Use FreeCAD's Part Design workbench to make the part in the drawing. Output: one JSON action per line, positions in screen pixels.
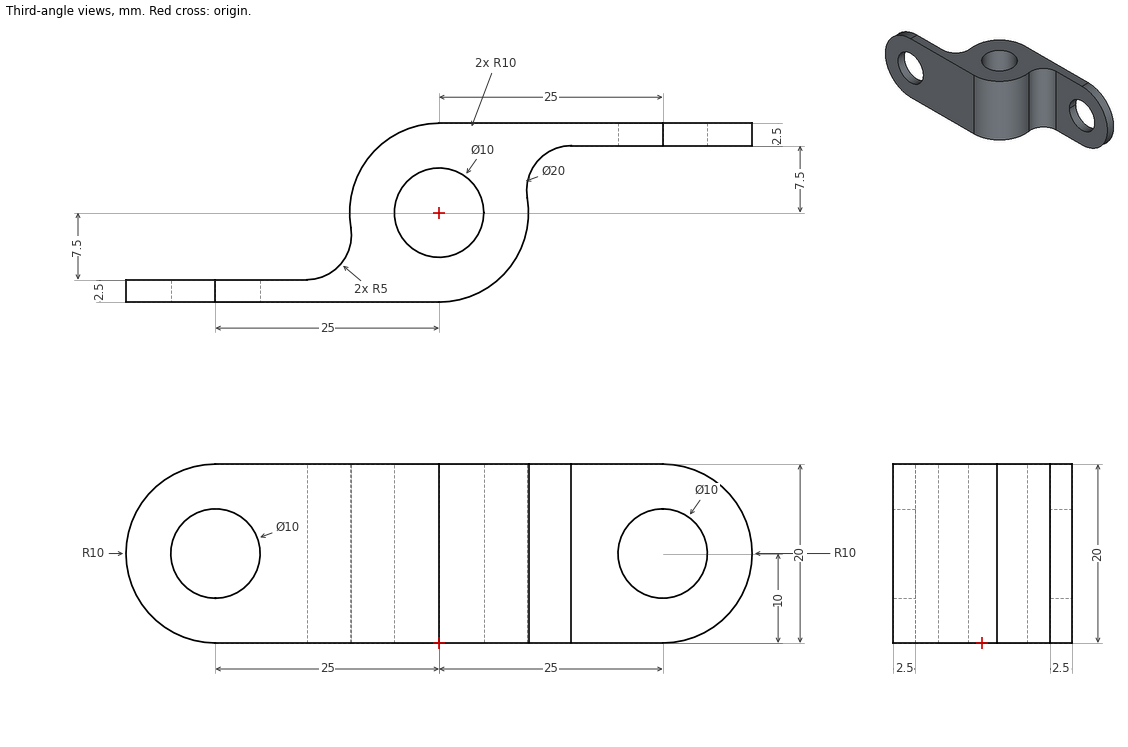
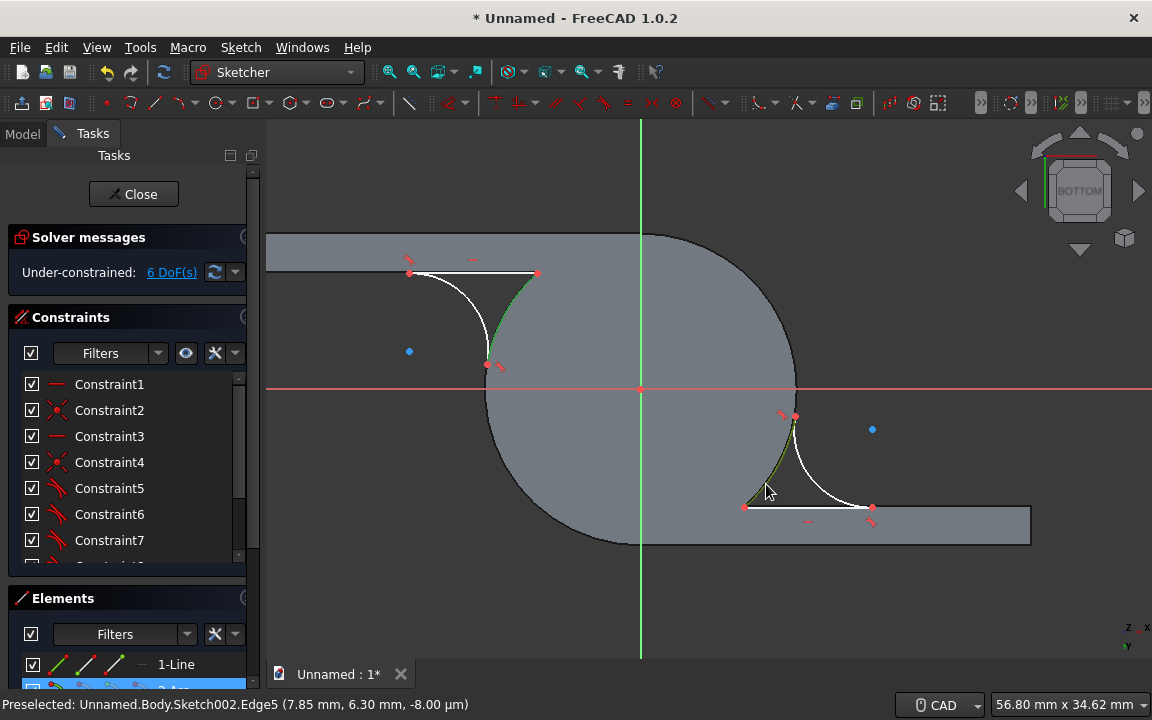
{"action": "key", "text": "e"}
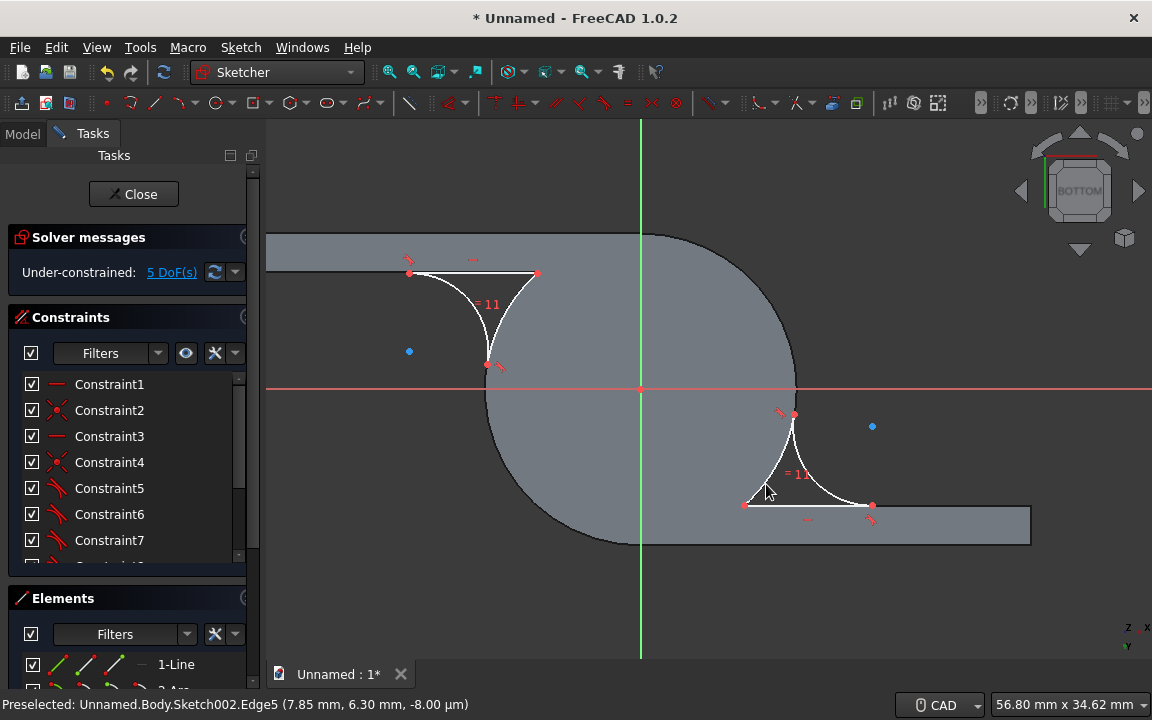
{"action": "left_click", "coordinate": [483, 324]}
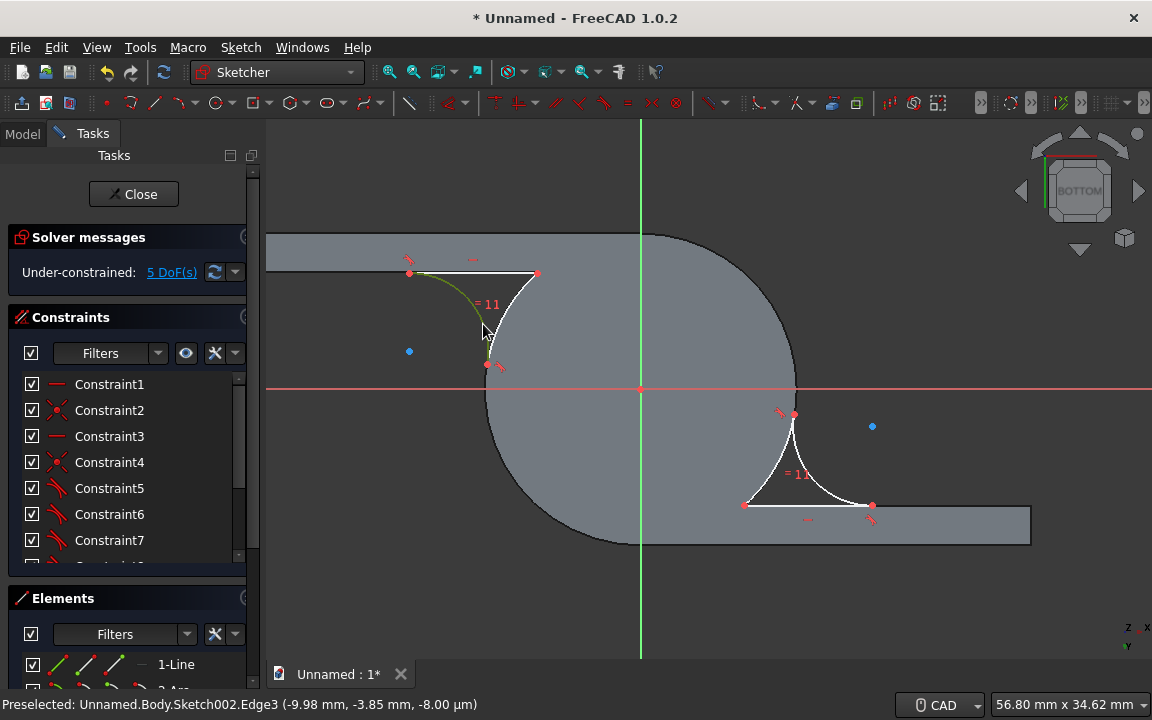
{"action": "left_click", "coordinate": [798, 455]}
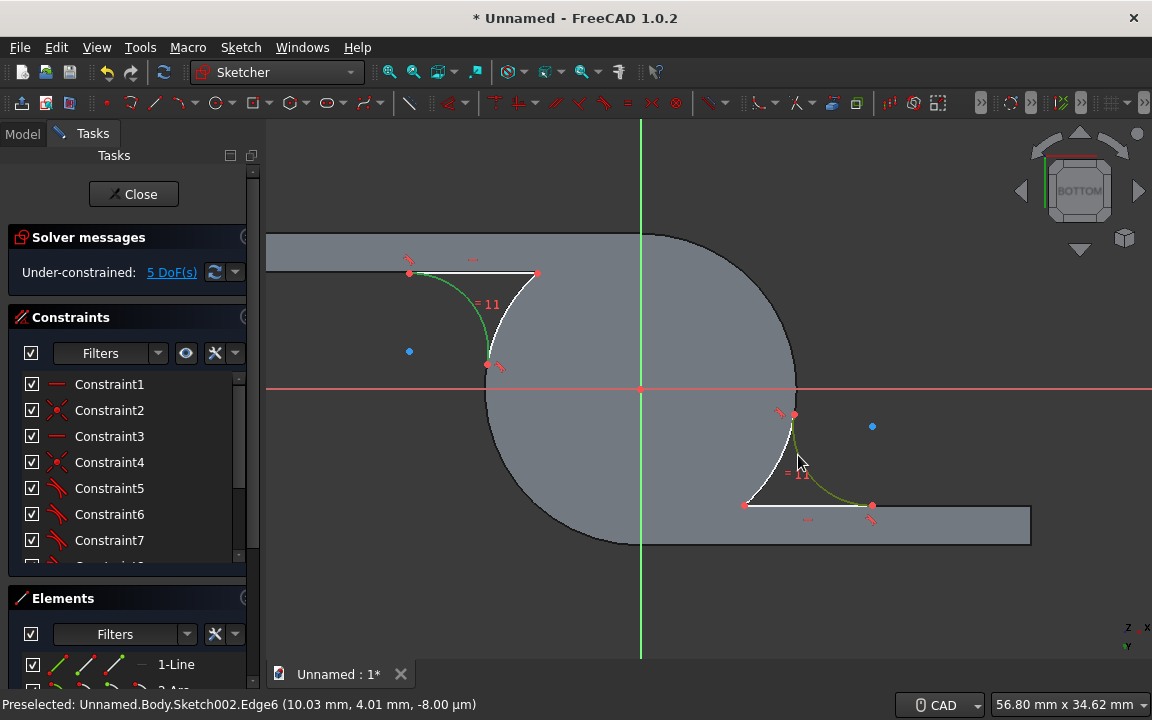
{"action": "key", "text": "e"}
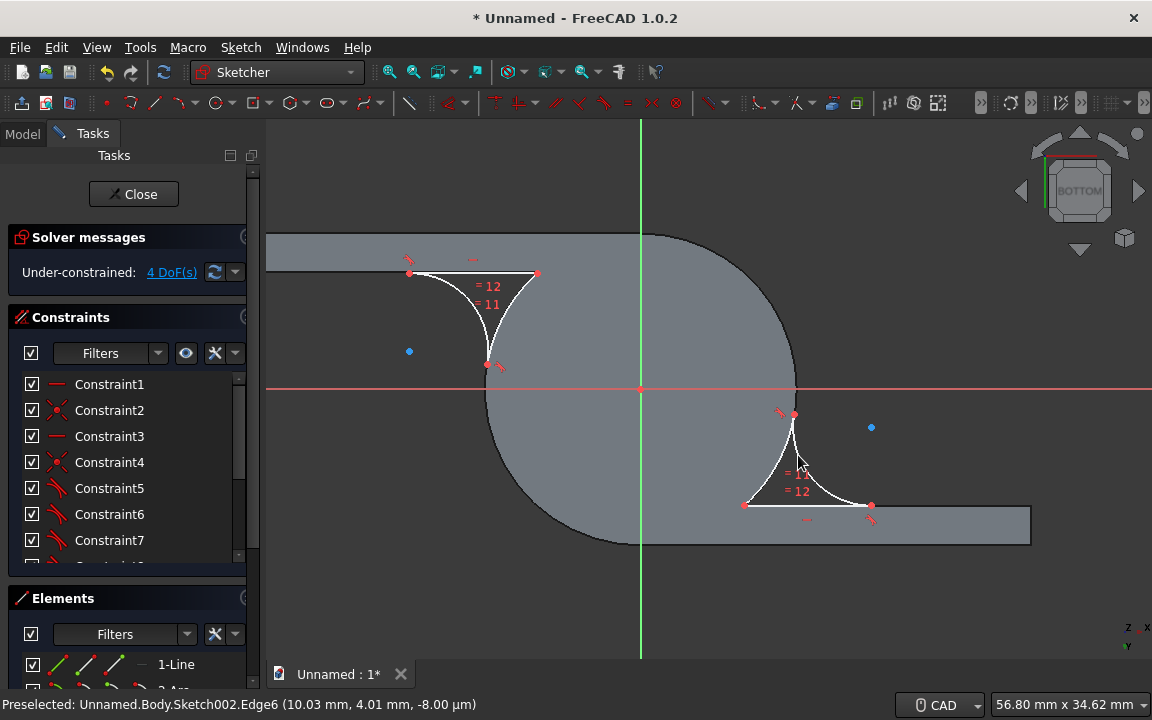
{"action": "left_click", "coordinate": [448, 104]}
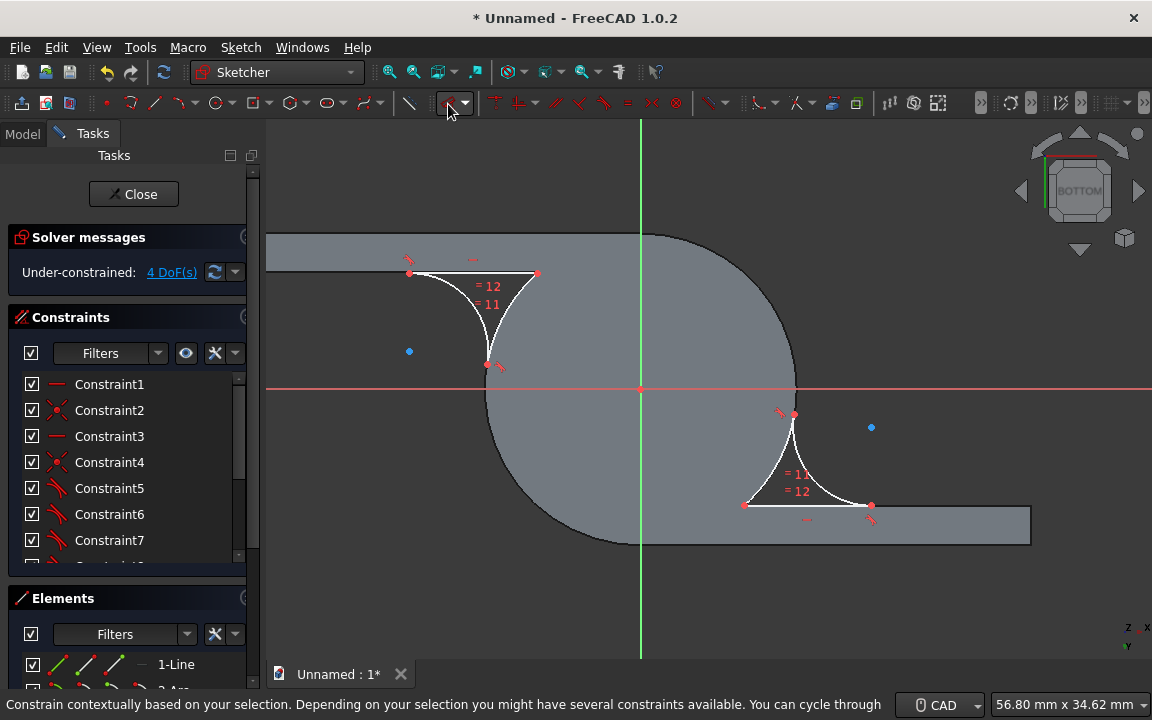
{"action": "left_click", "coordinate": [516, 297]}
{"action": "left_click", "coordinate": [562, 219]}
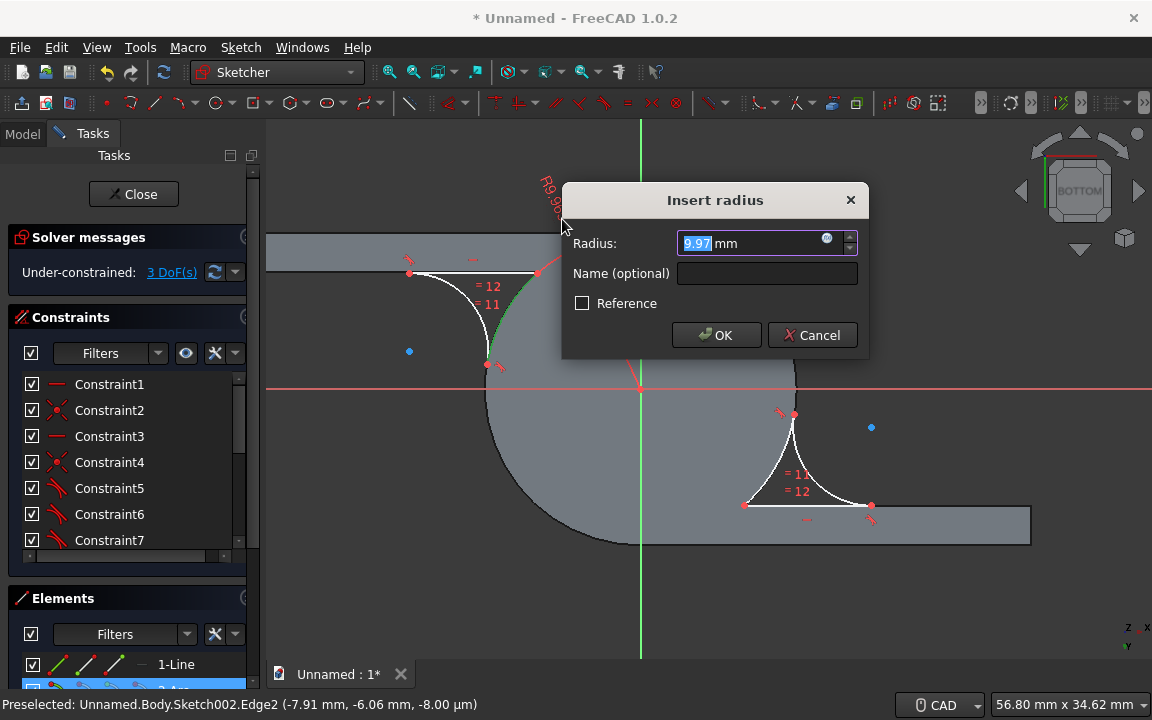
{"action": "type", "text": "10"}
{"action": "key", "text": "Return"}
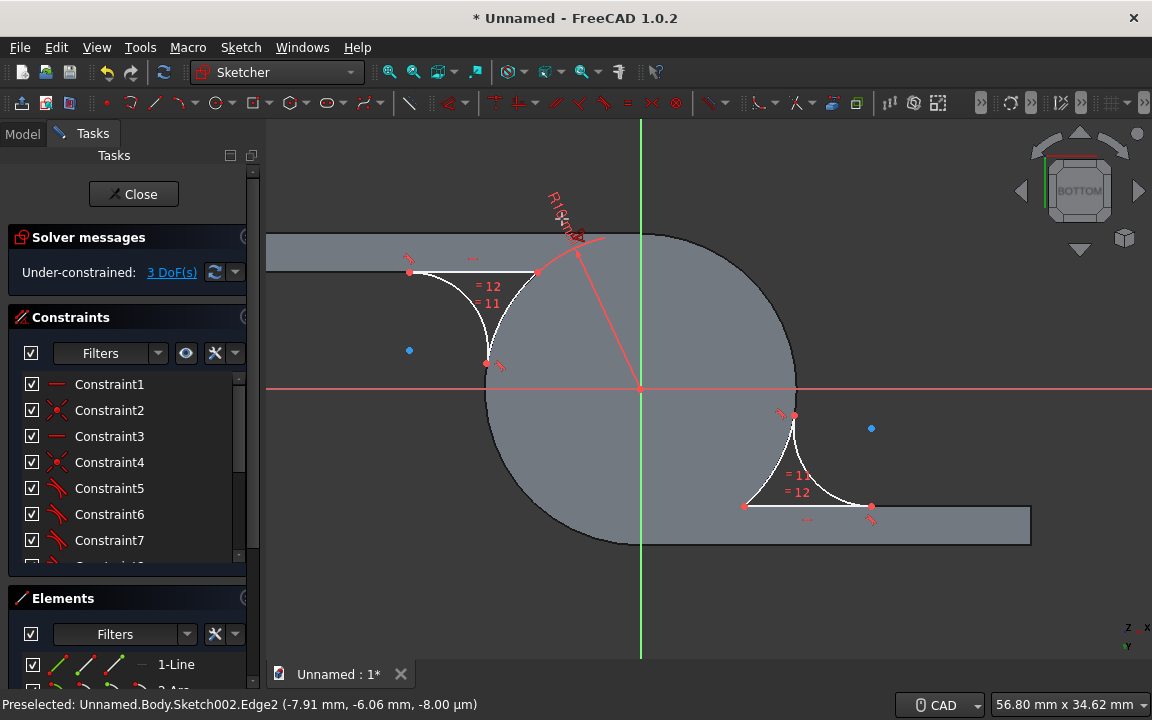
{"action": "left_click", "coordinate": [483, 323]}
{"action": "left_click", "coordinate": [519, 366]}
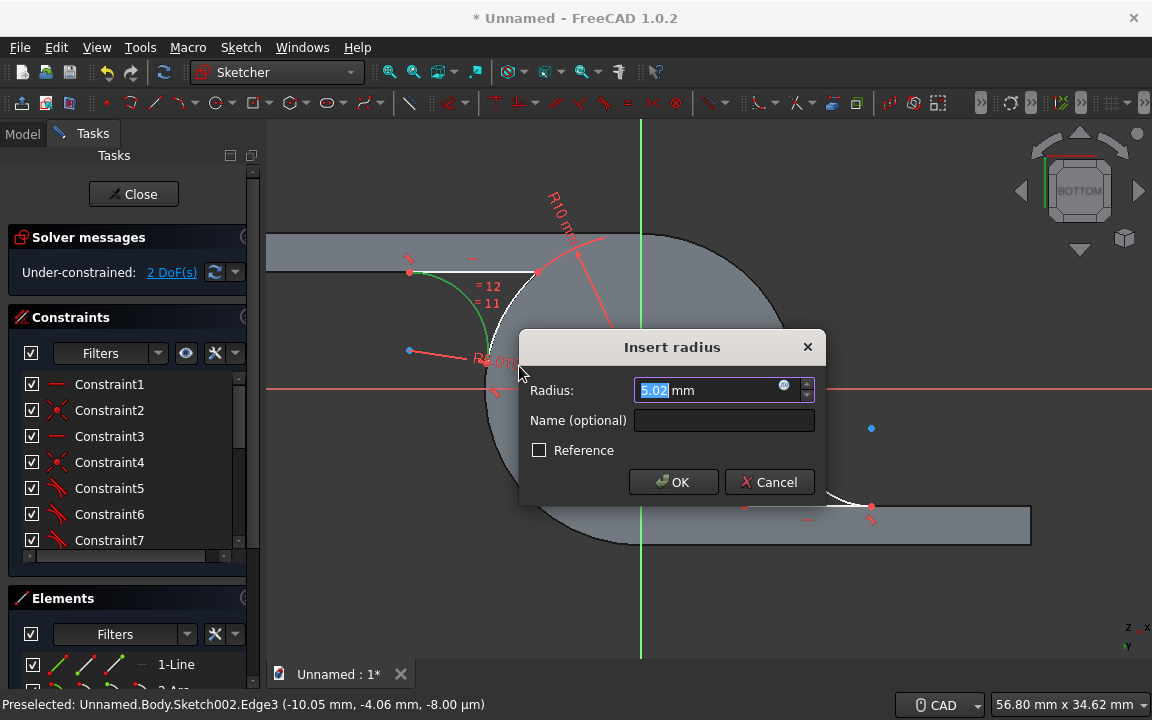
{"action": "type", "text": "5"}
{"action": "key", "text": "Return"}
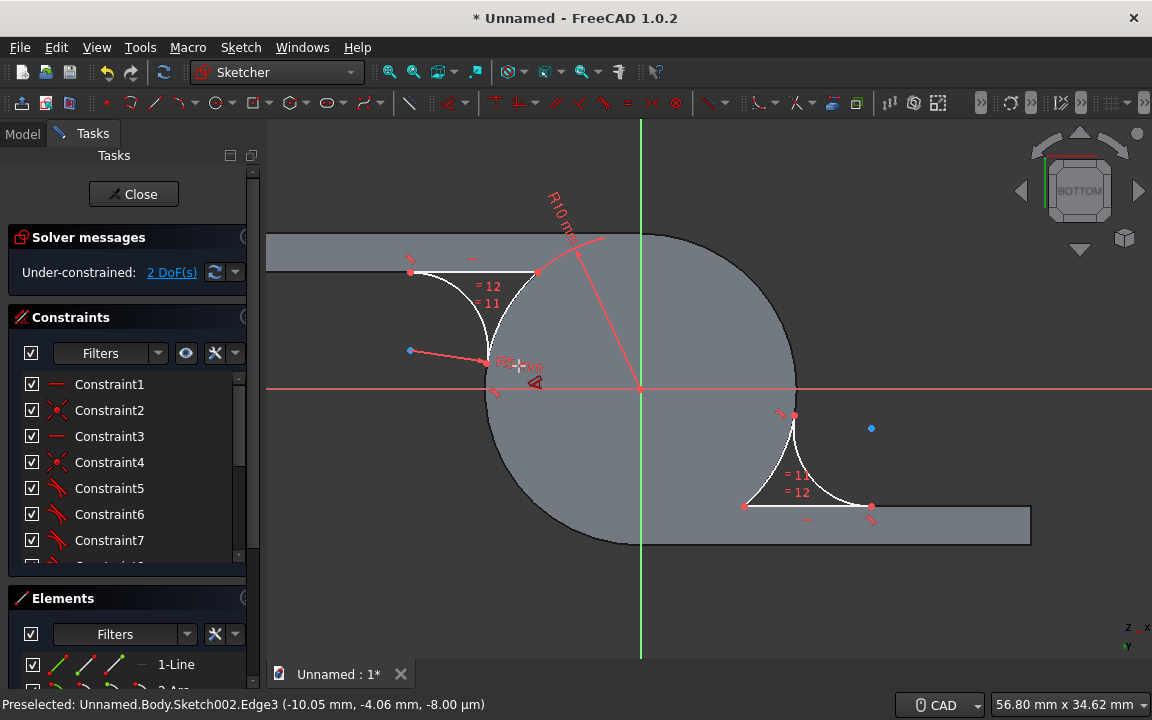
{"action": "left_click", "coordinate": [410, 272]}
{"action": "left_click", "coordinate": [376, 331]}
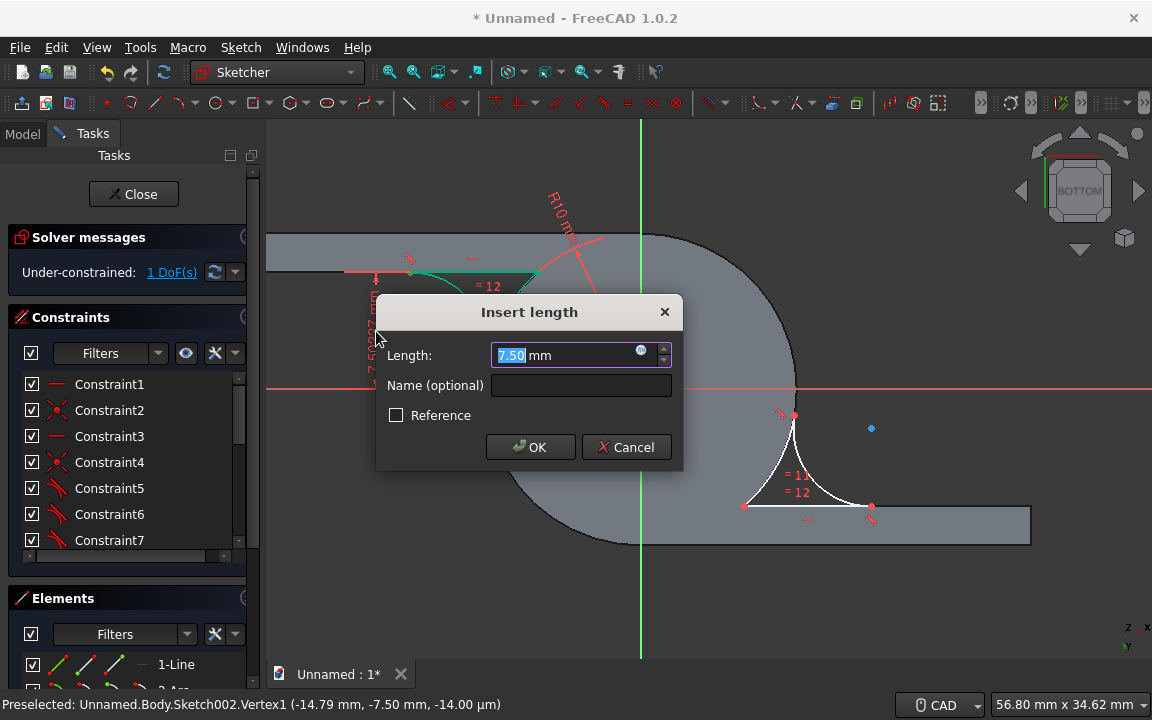
{"action": "type", "text": "7.5"}
{"action": "key", "text": "Return"}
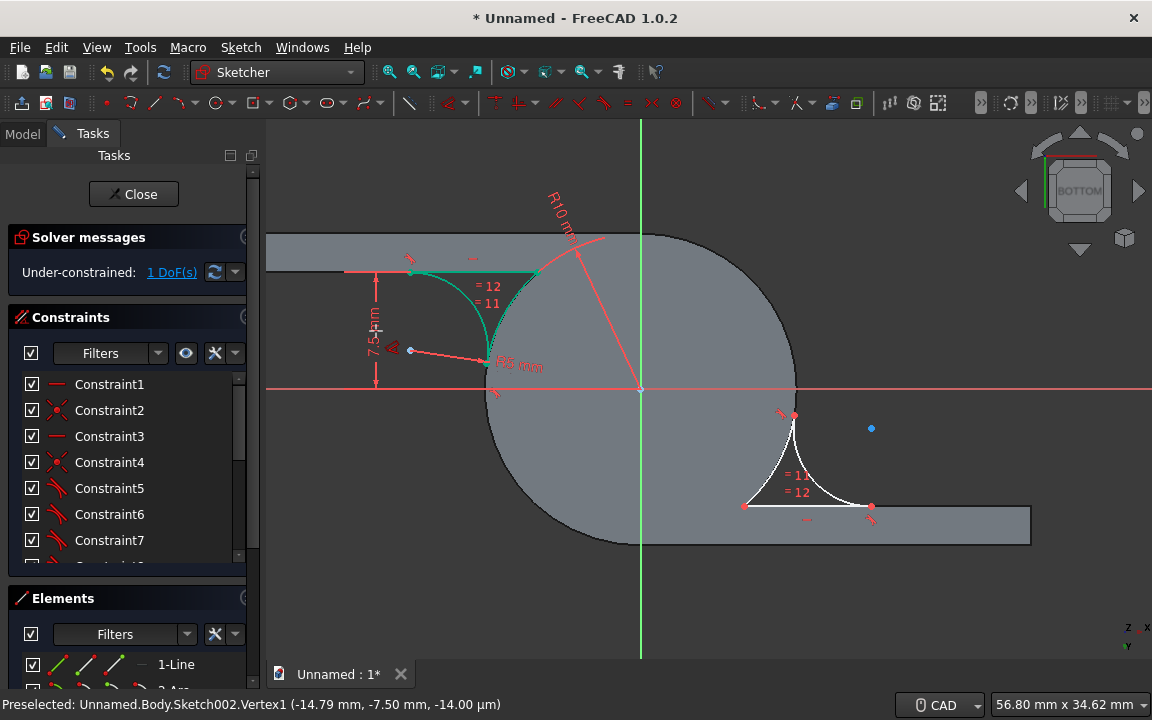
{"action": "left_click", "coordinate": [872, 506]}
{"action": "left_click", "coordinate": [906, 448]}